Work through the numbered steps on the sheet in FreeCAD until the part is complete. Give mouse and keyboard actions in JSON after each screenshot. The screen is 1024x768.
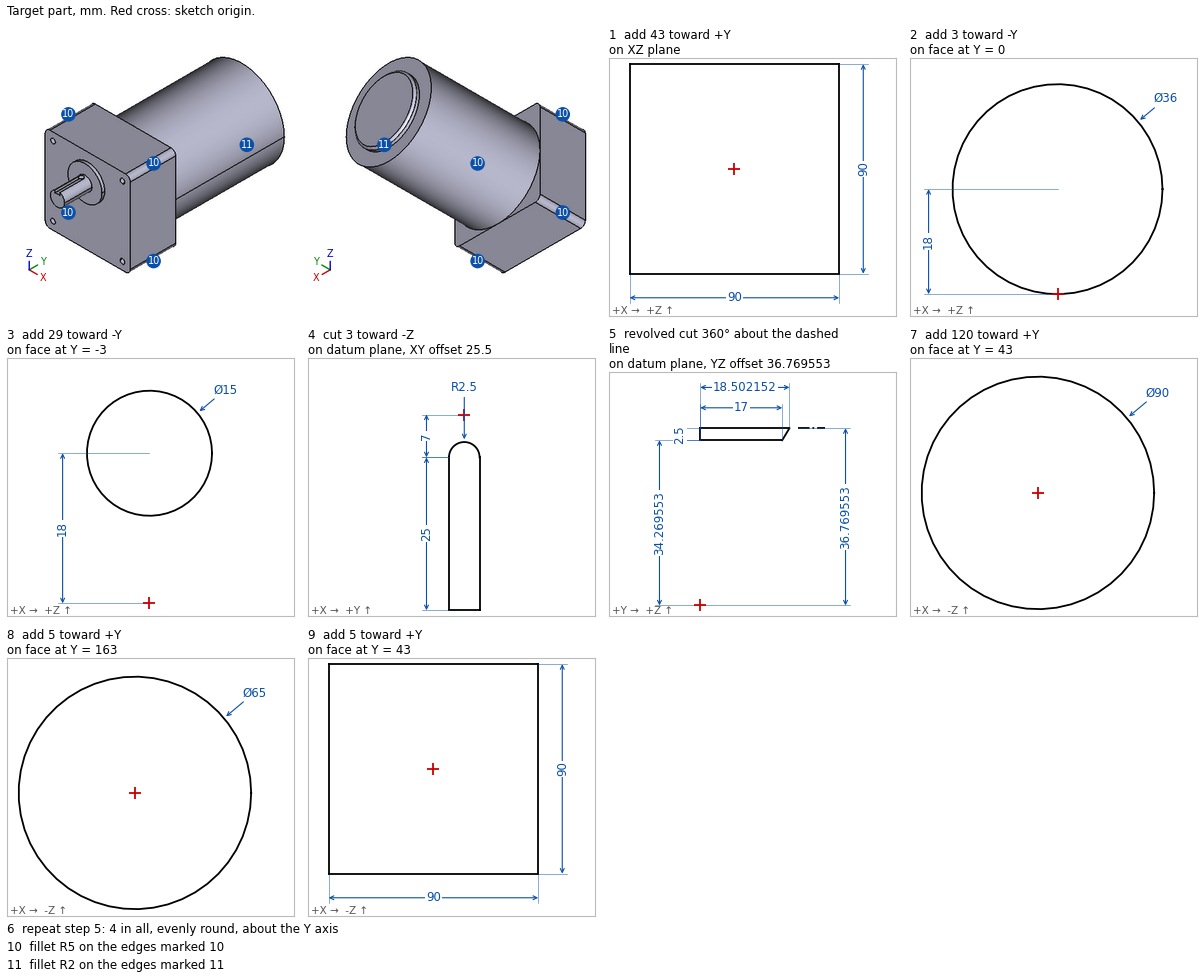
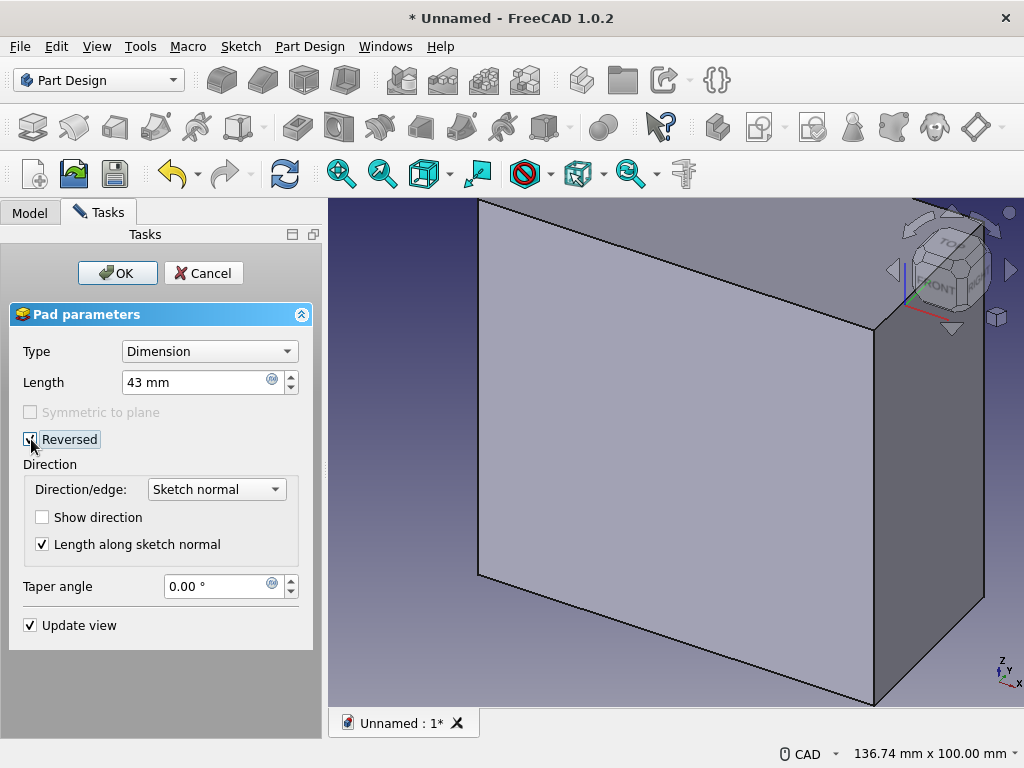
{"action": "left_click", "coordinate": [118, 273]}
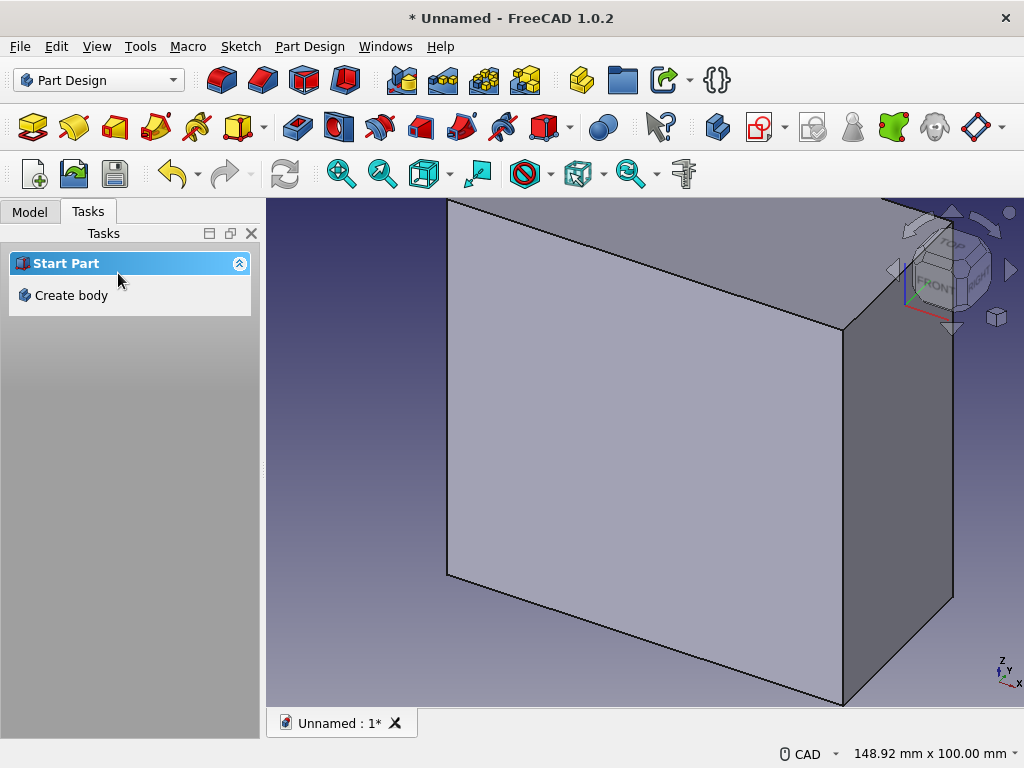
{"action": "left_click", "coordinate": [342, 174]}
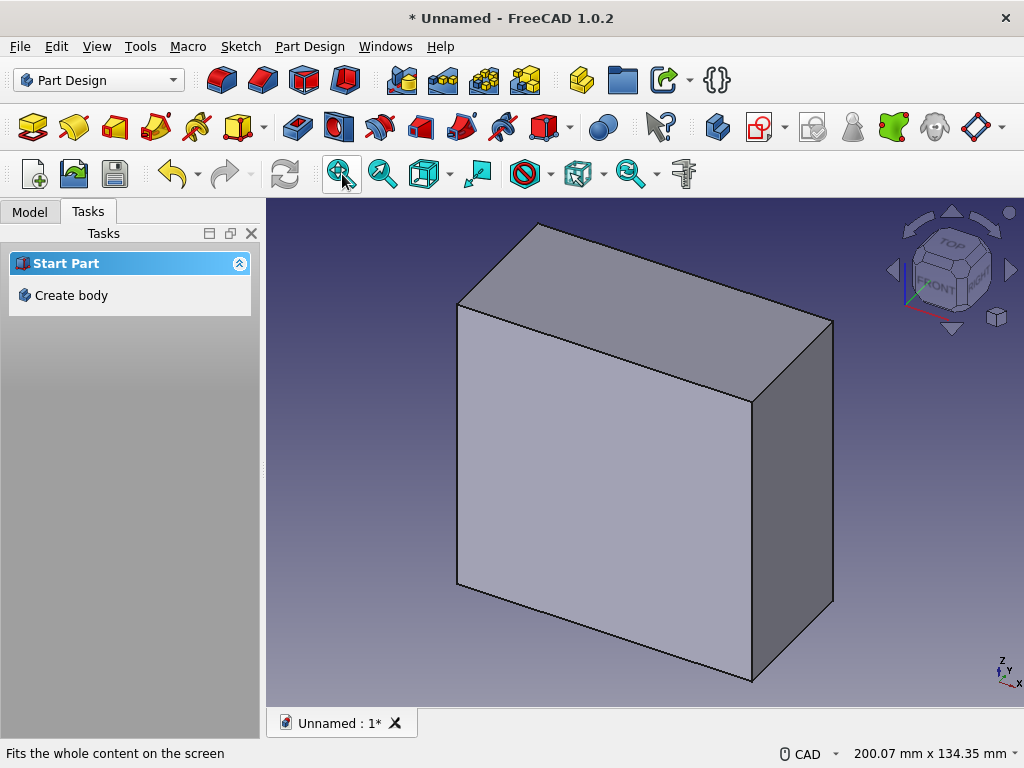
{"action": "left_click", "coordinate": [604, 492]}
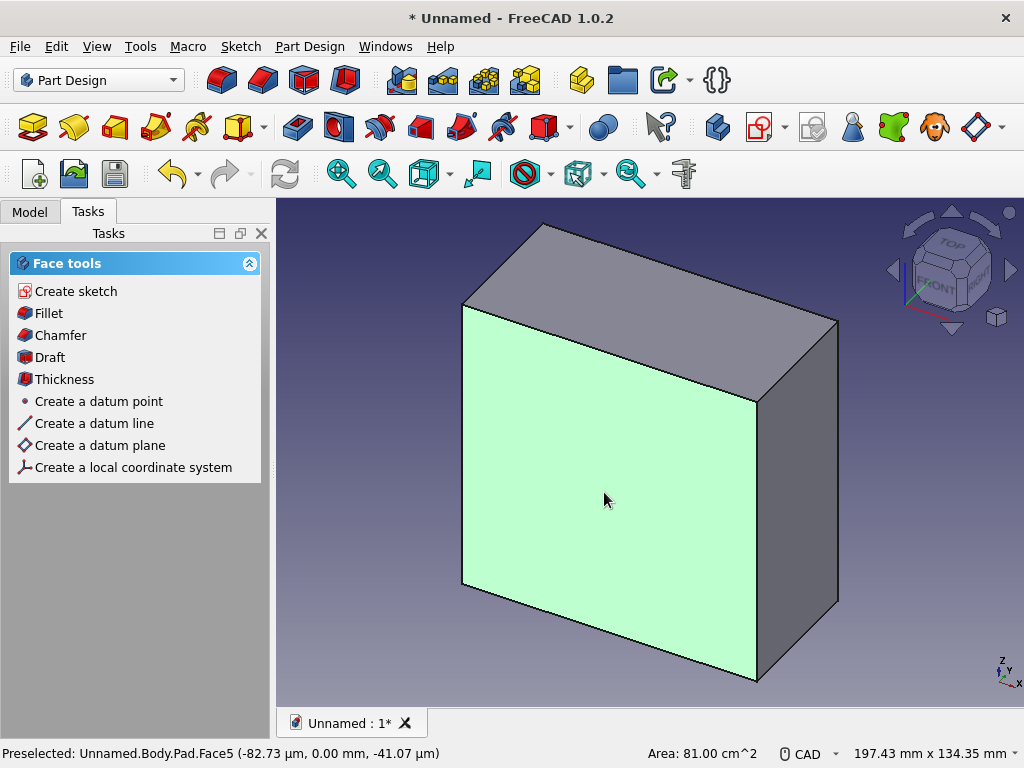
{"action": "left_click", "coordinate": [758, 128]}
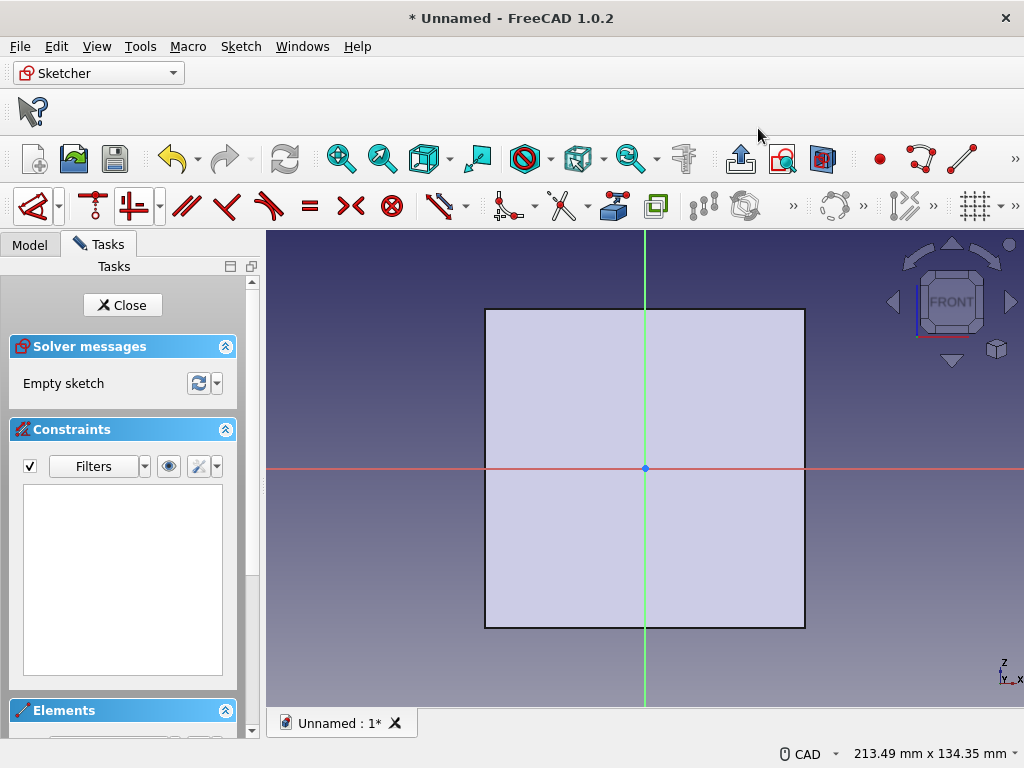
{"action": "scroll", "coordinate": [701, 352], "scroll_direction": "up", "scroll_amount": 4}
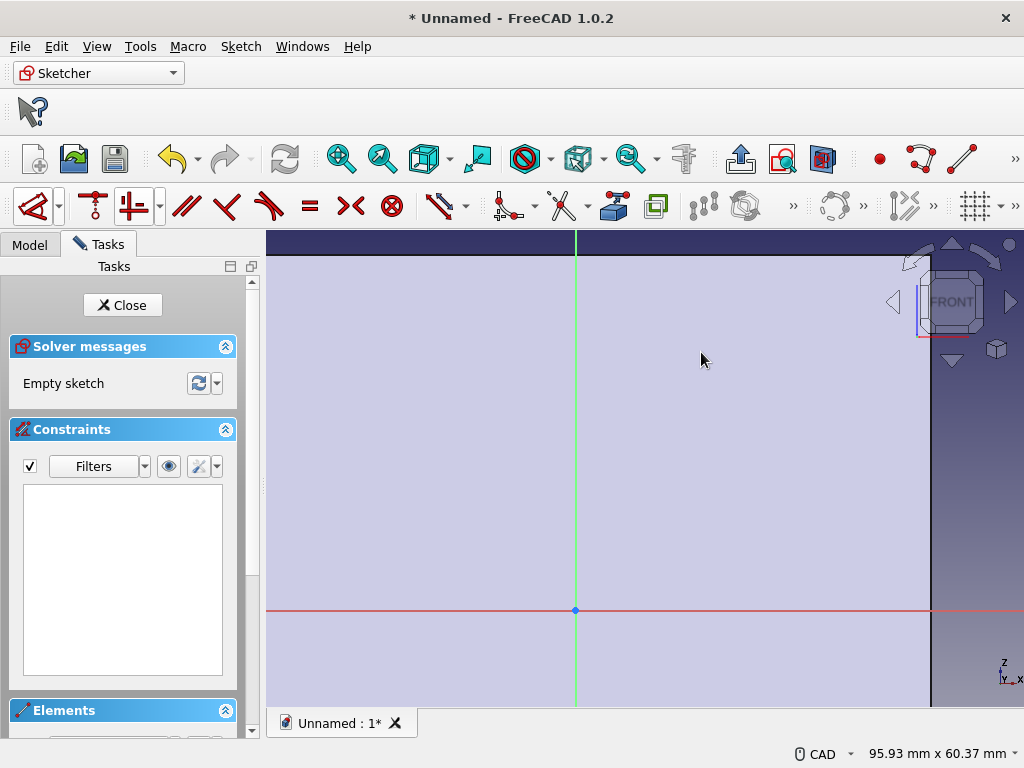
{"action": "key", "text": "g c"}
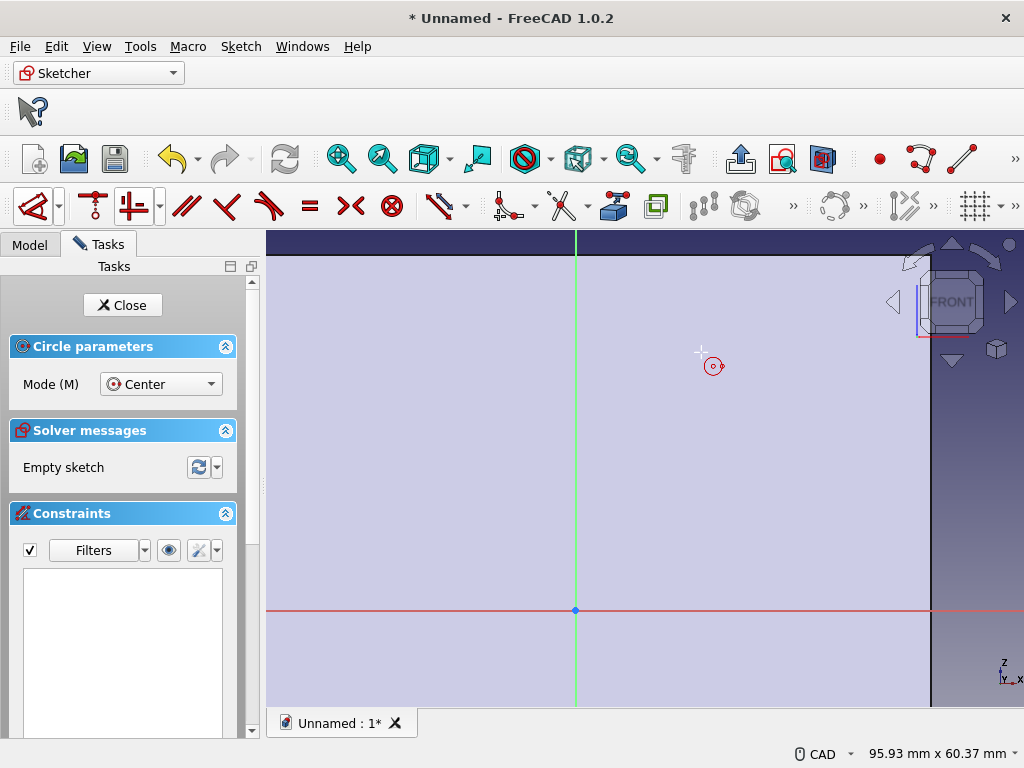
{"action": "left_click", "coordinate": [576, 469]}
{"action": "mouse_move", "coordinate": [676, 368]}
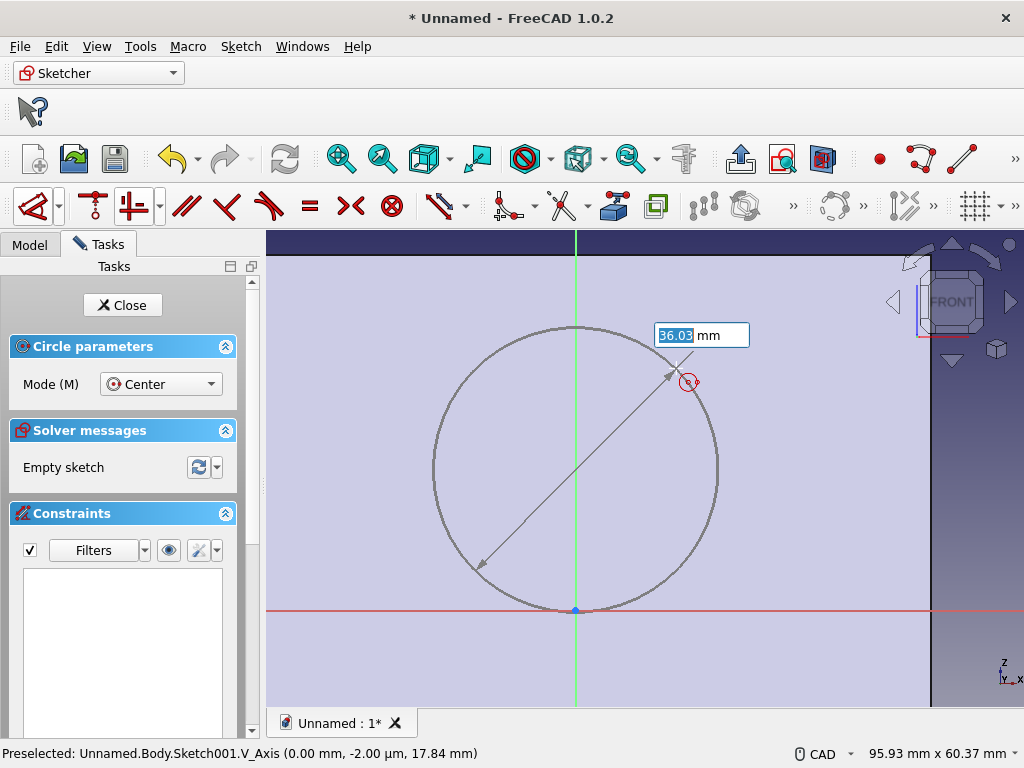
{"action": "type", "text": "36"}
{"action": "key", "text": "Return"}
{"action": "key", "text": "Escape"}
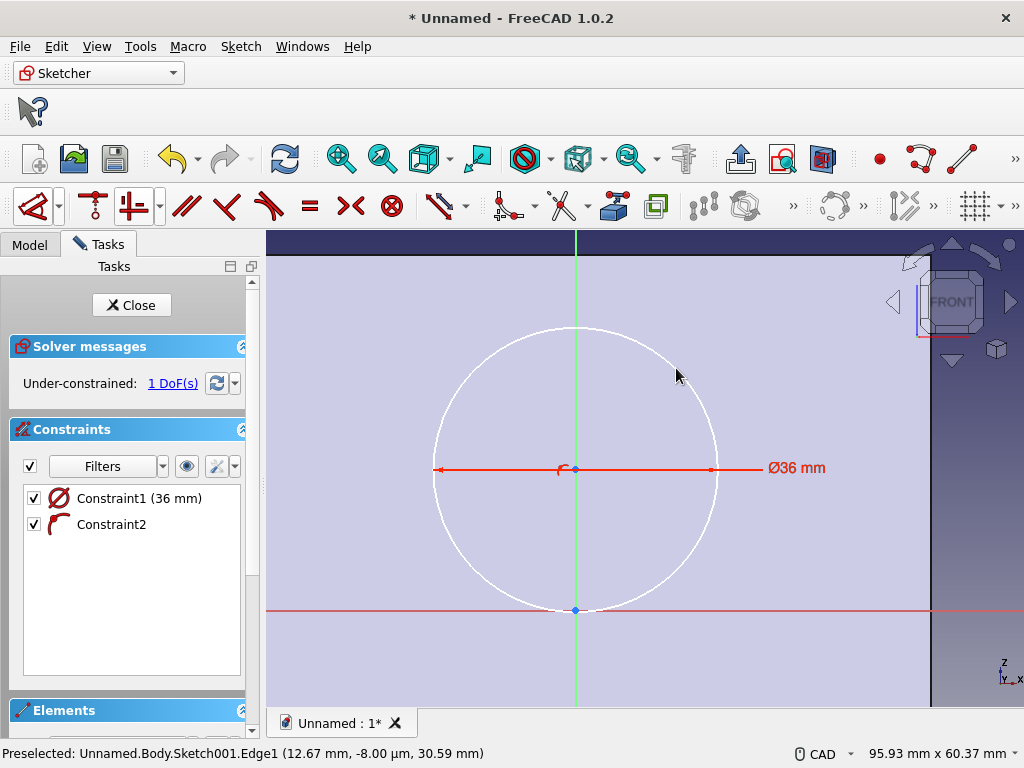
{"action": "left_click", "coordinate": [576, 470]}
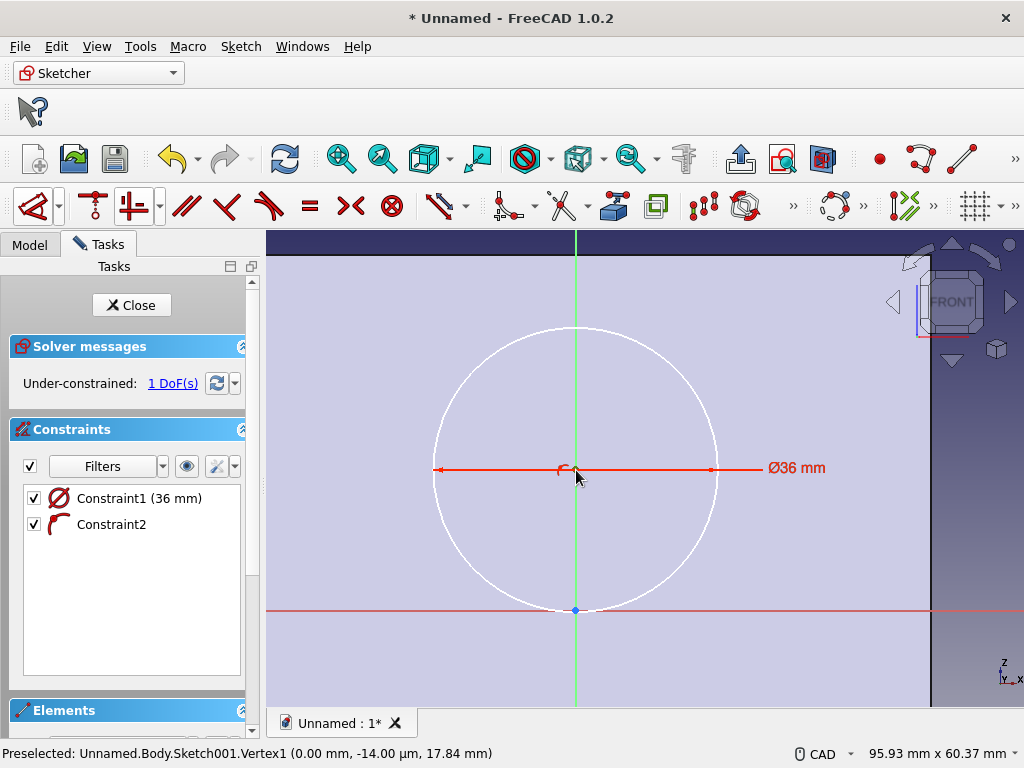
{"action": "key", "text": "i"}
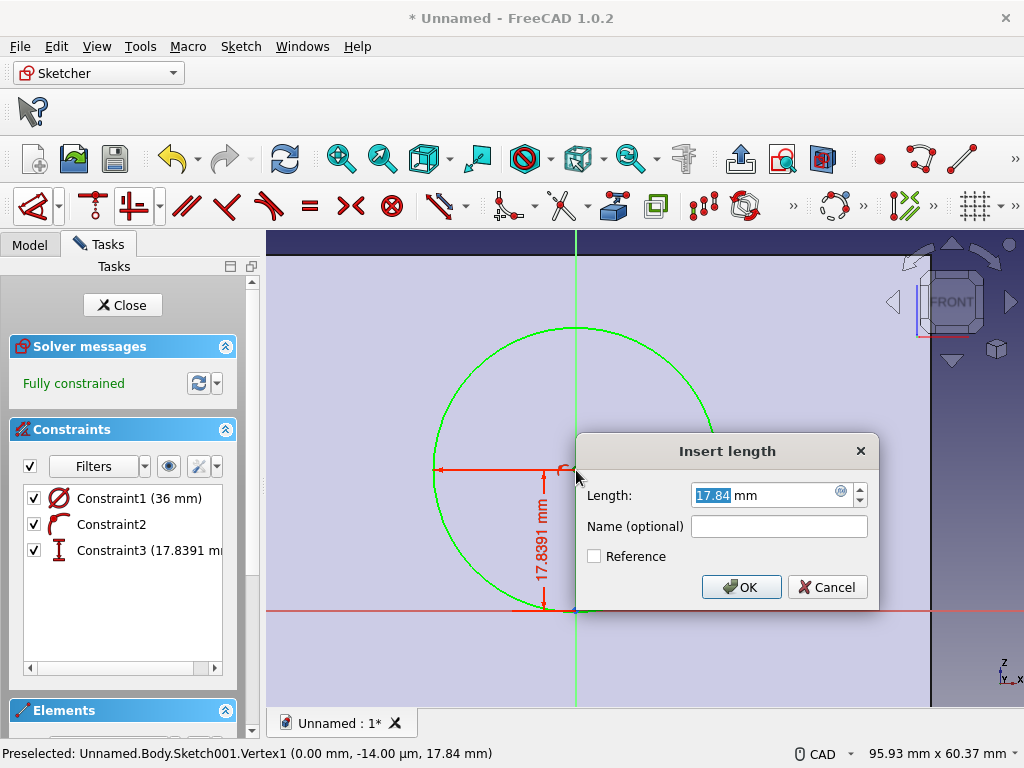
{"action": "type", "text": "18"}
{"action": "key", "text": "Return"}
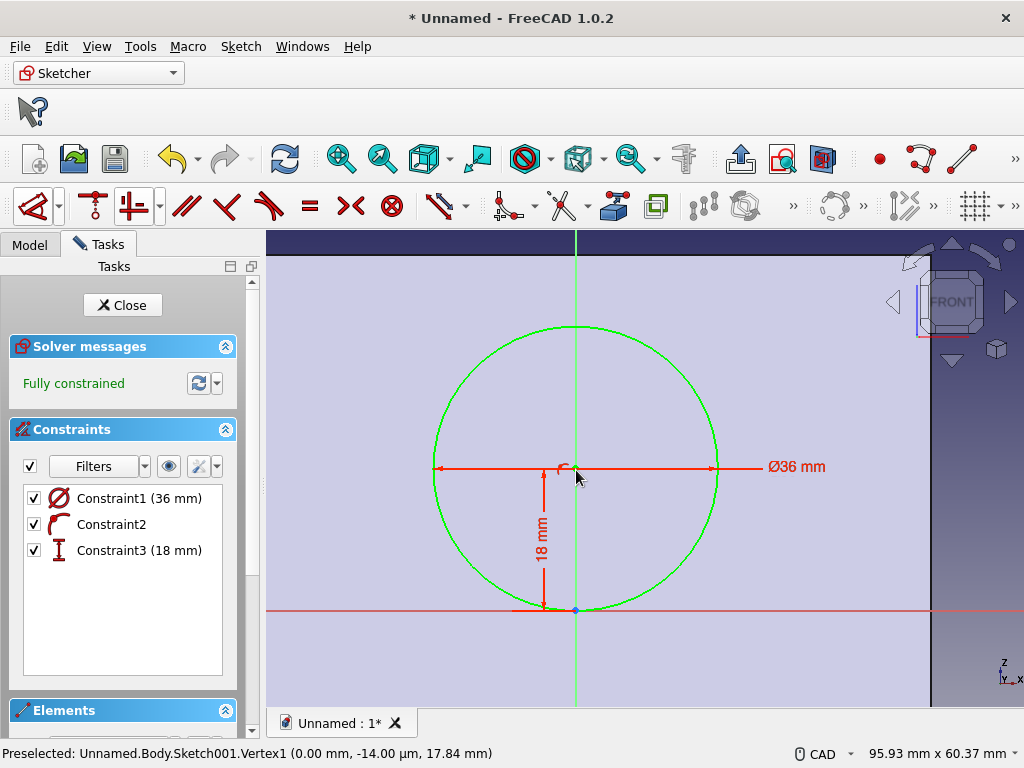
{"action": "left_click", "coordinate": [123, 305]}